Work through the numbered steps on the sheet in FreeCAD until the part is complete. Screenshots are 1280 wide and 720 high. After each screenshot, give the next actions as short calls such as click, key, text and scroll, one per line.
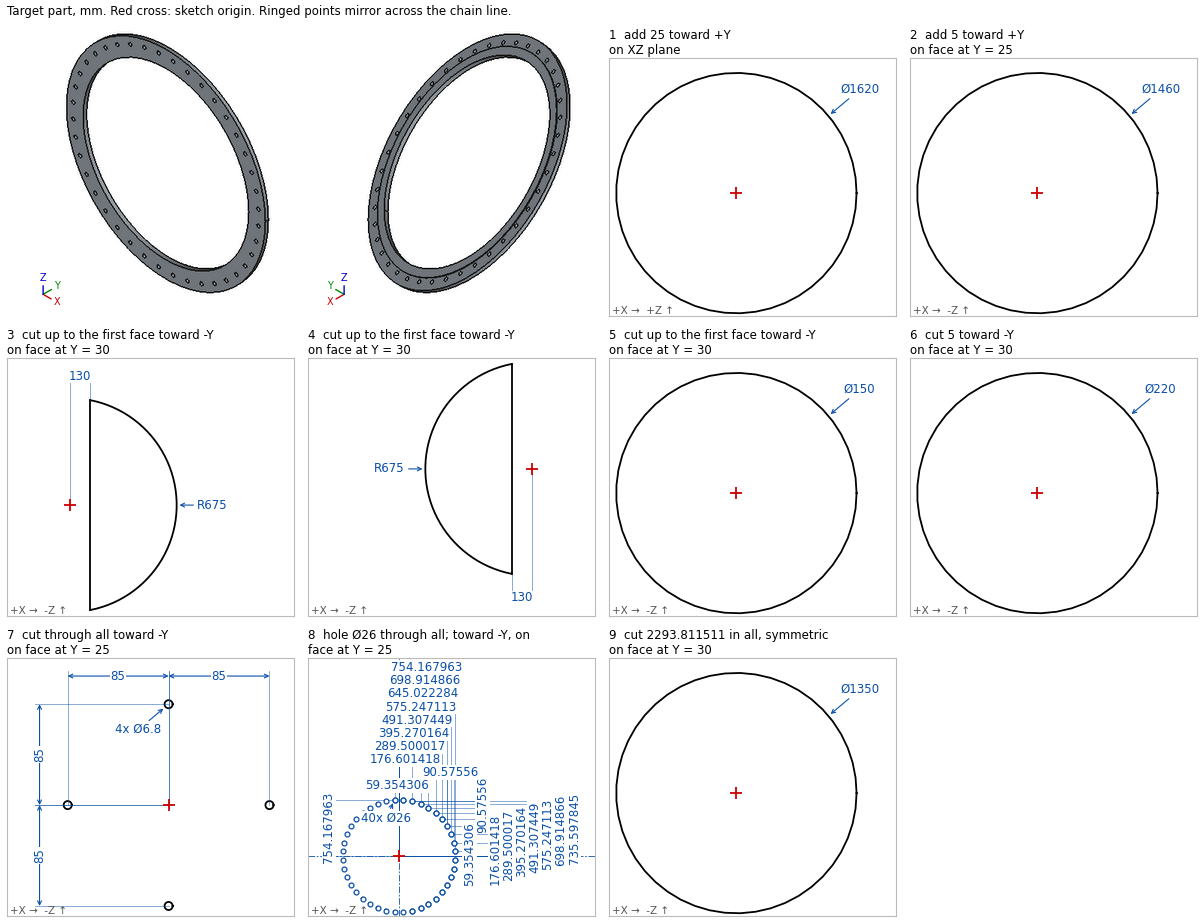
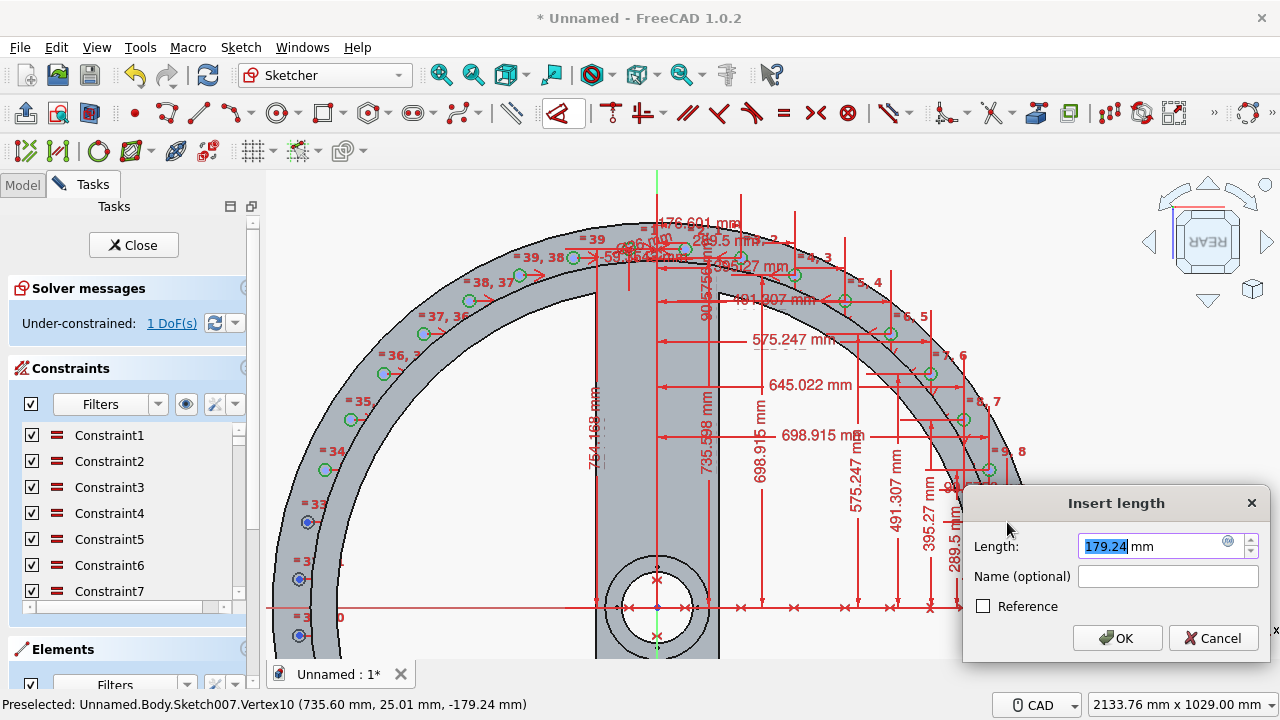
text(176.601418)
key(Return)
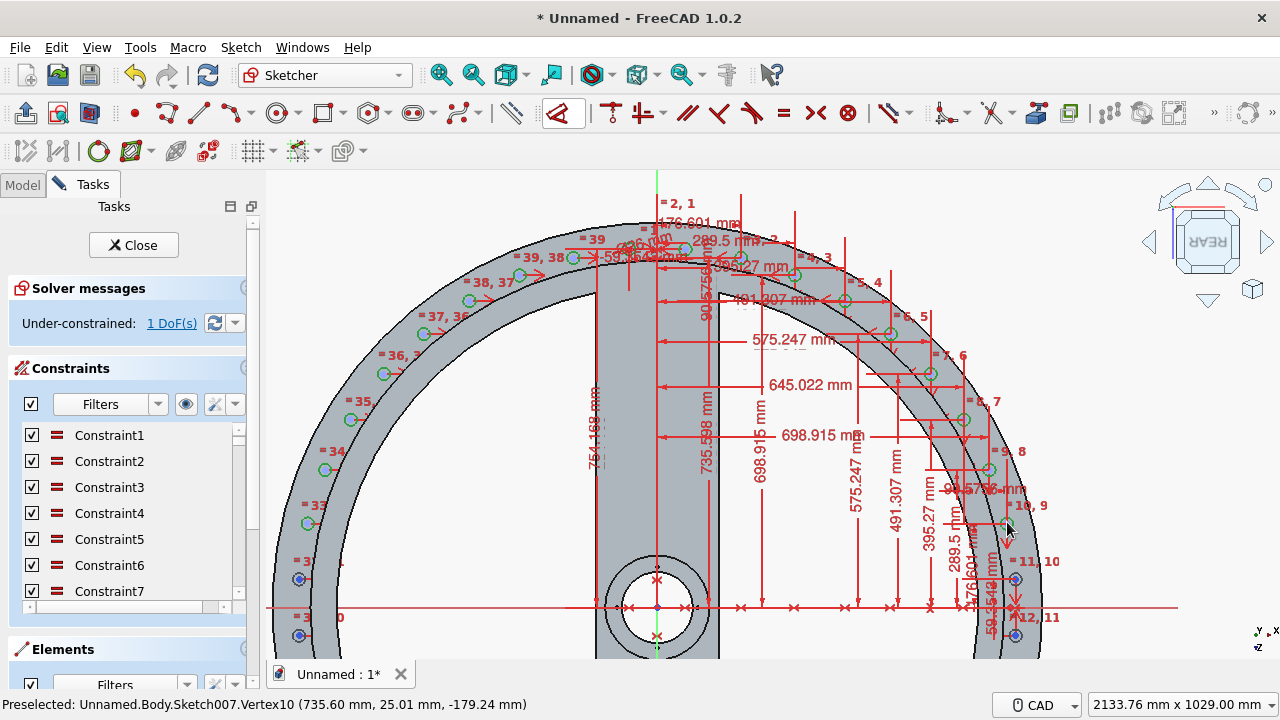
click(1016, 579)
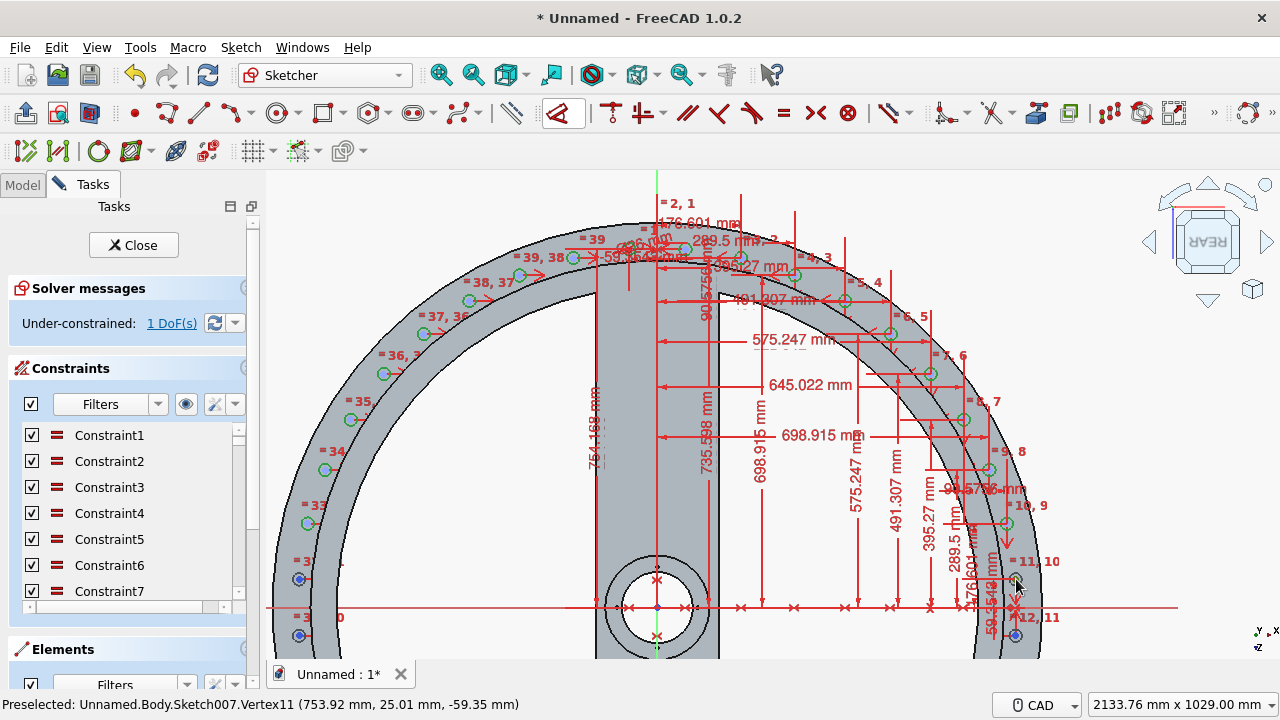
click(580, 114)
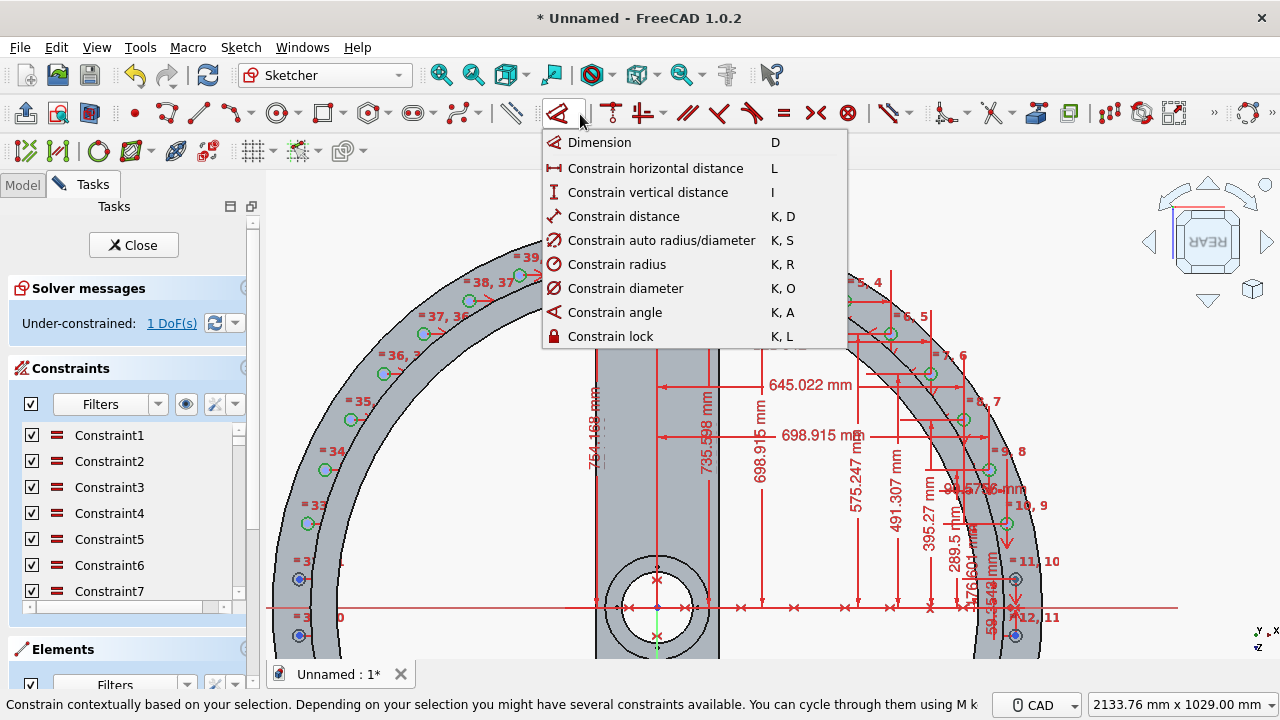
click(695, 168)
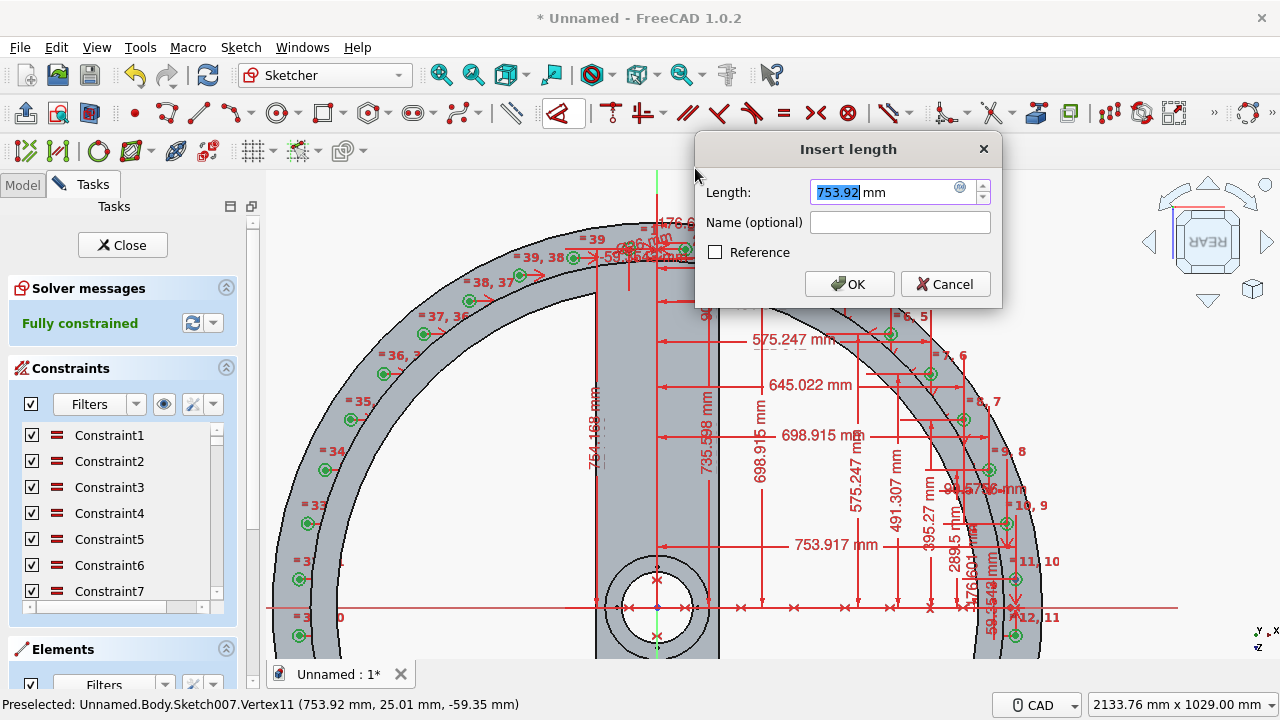
text(754.167963)
key(Return)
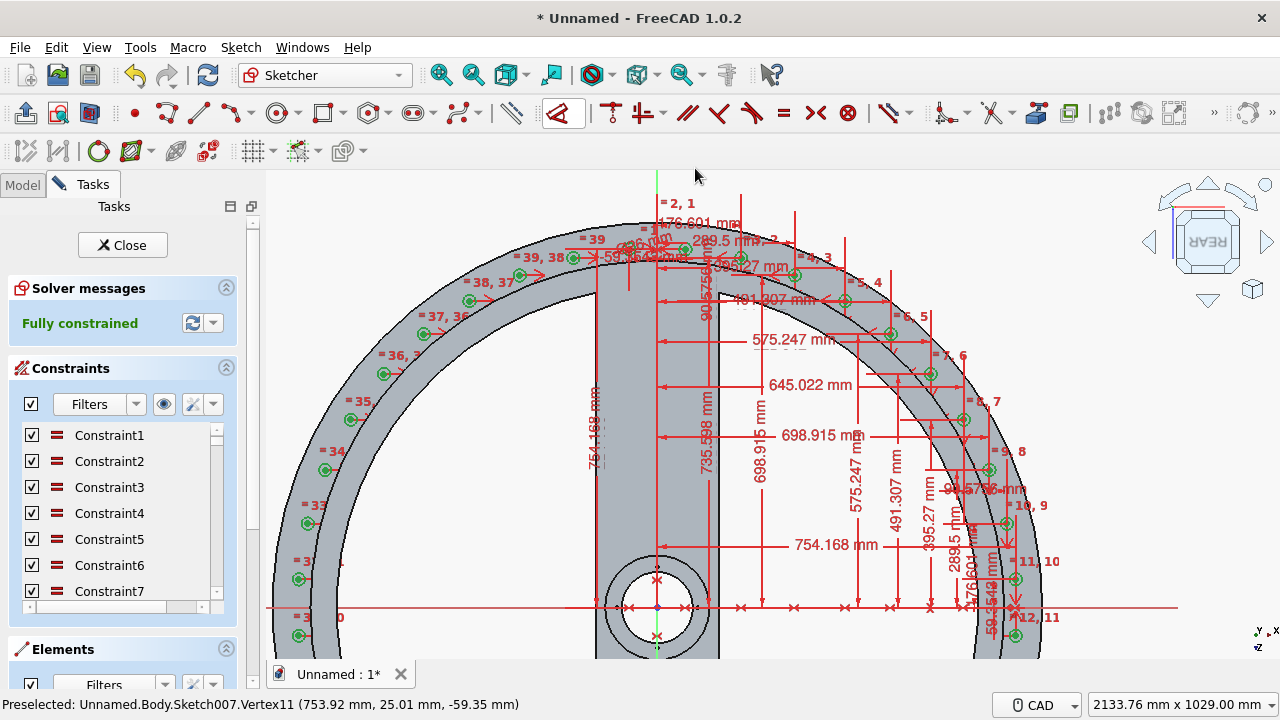
click(123, 245)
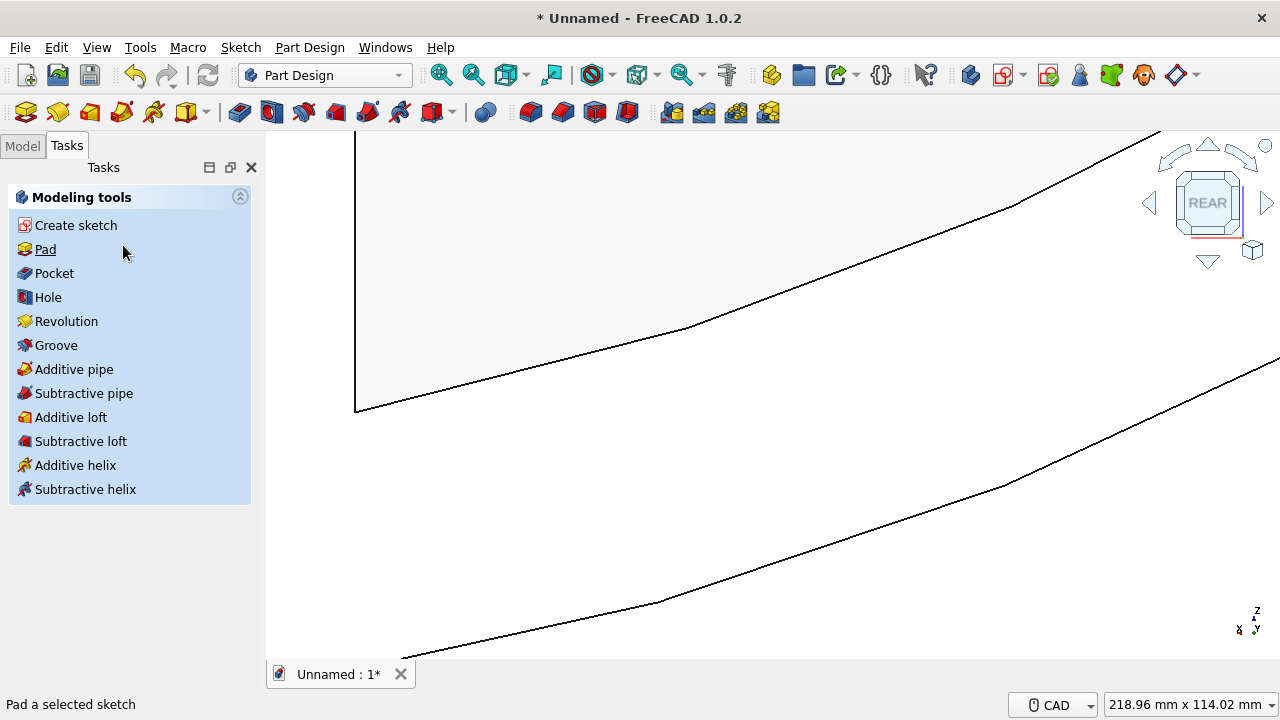
click(272, 112)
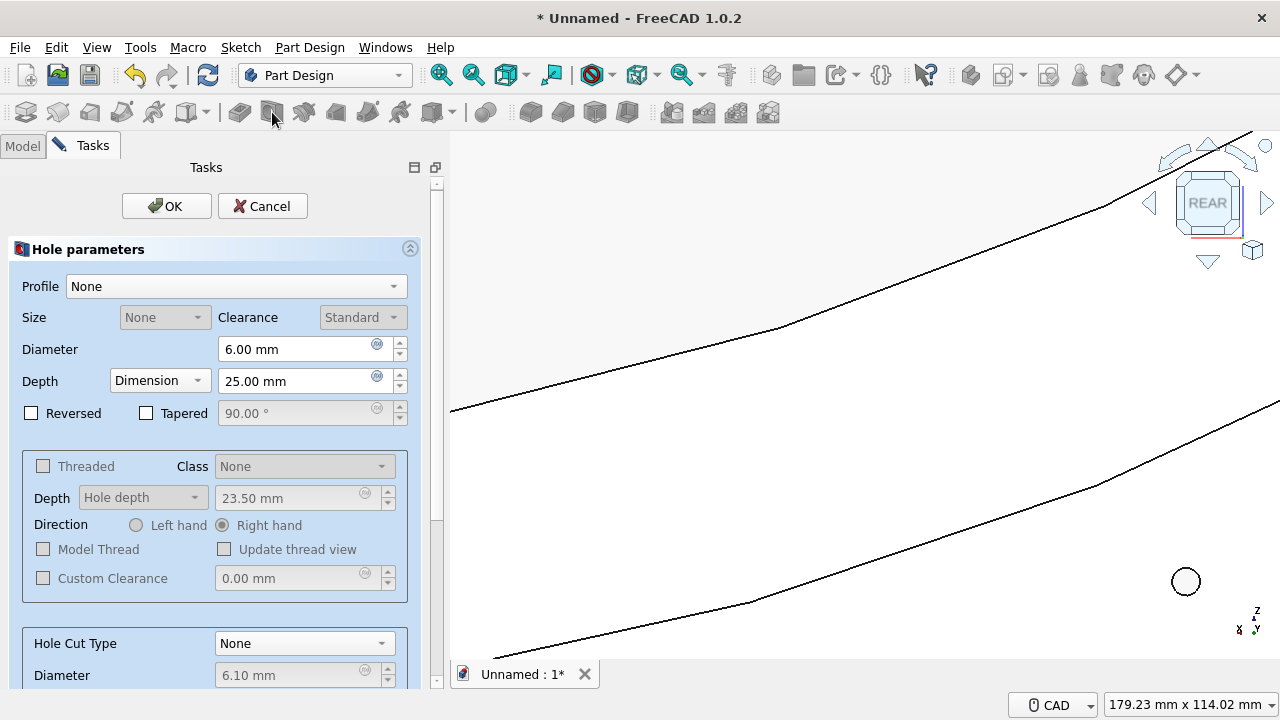
triple_click(305, 349)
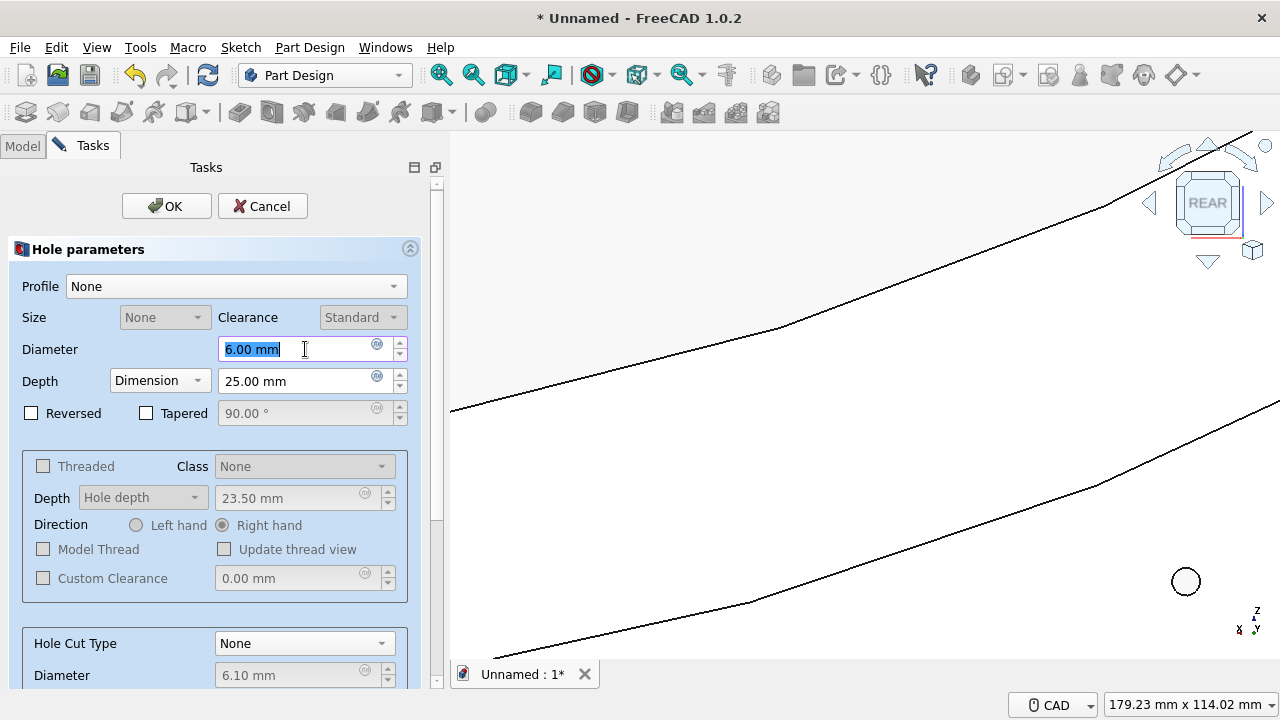
text(26)
key(Tab)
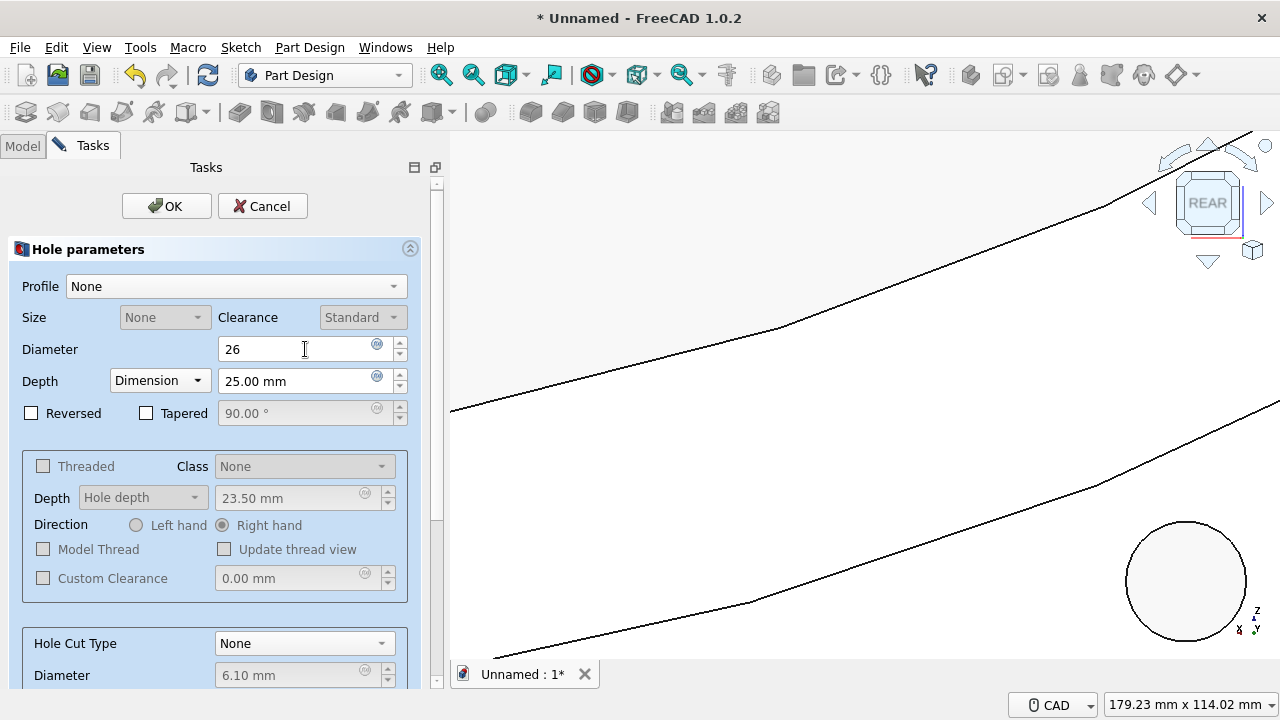
click(161, 380)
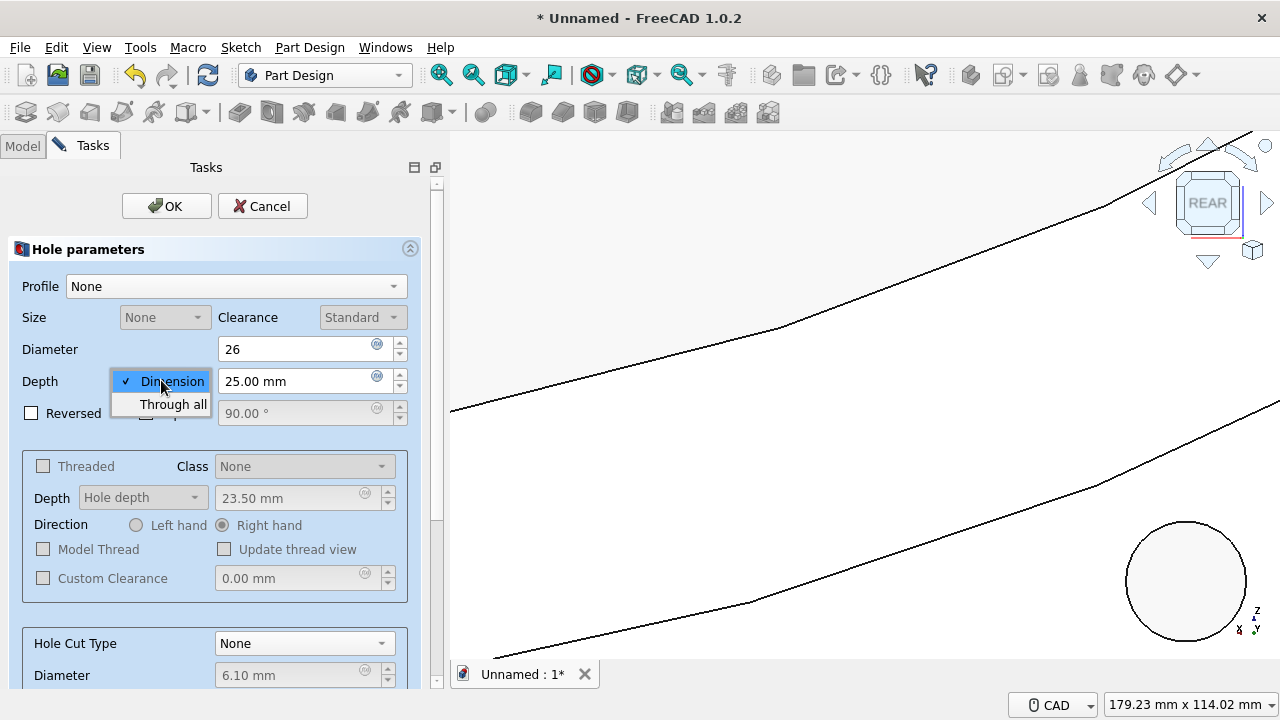
click(160, 404)